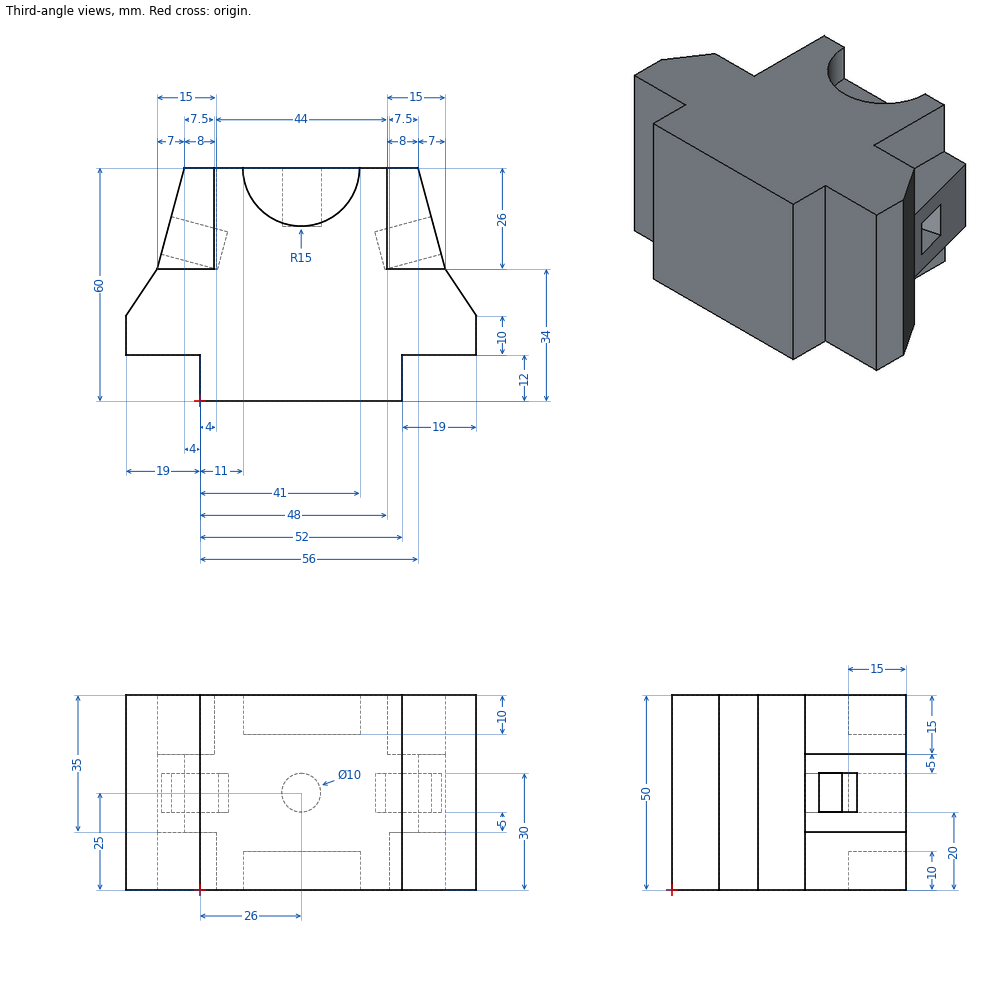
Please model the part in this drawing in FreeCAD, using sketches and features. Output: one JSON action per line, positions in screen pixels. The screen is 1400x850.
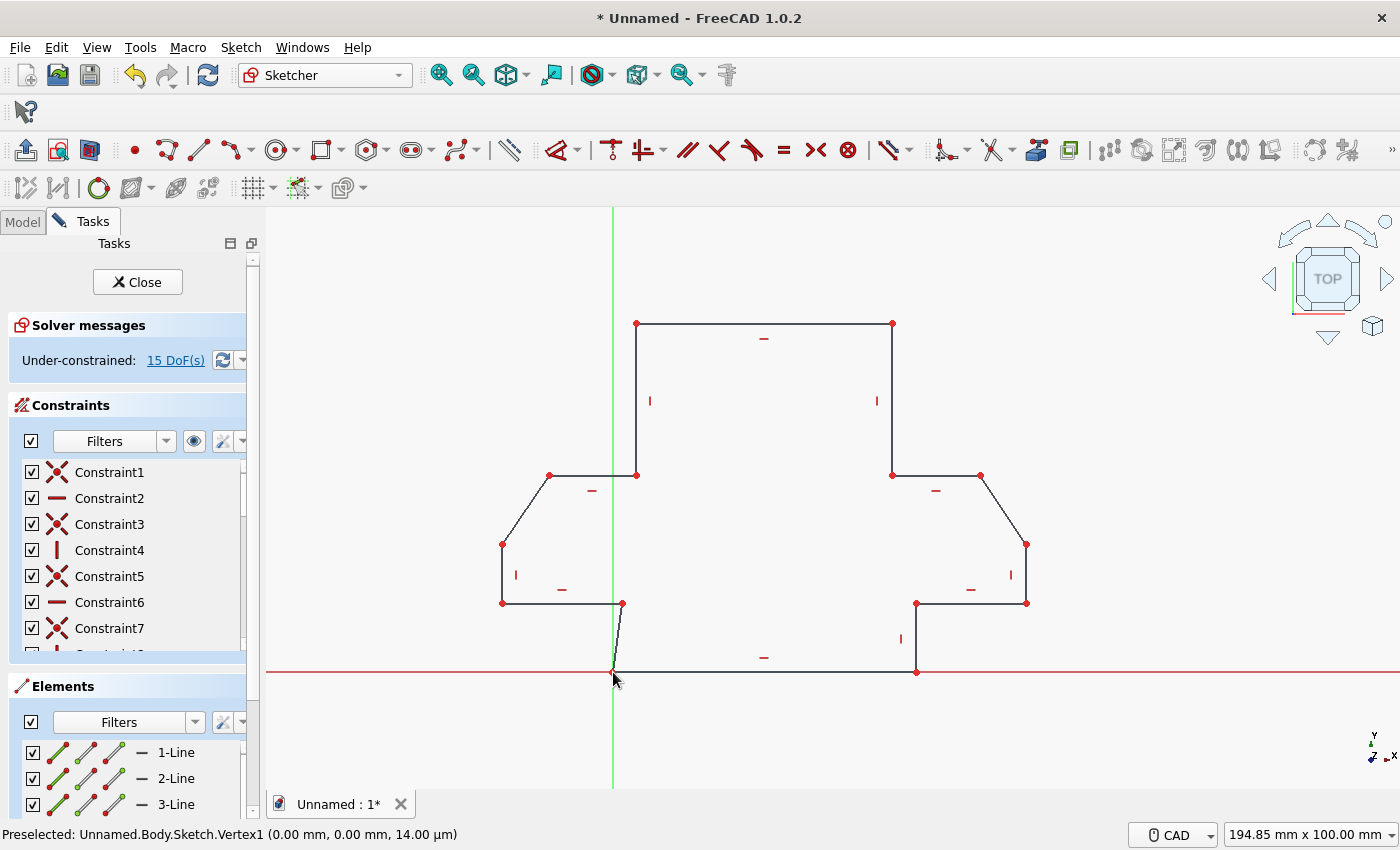
{"action": "left_click", "coordinate": [616, 652]}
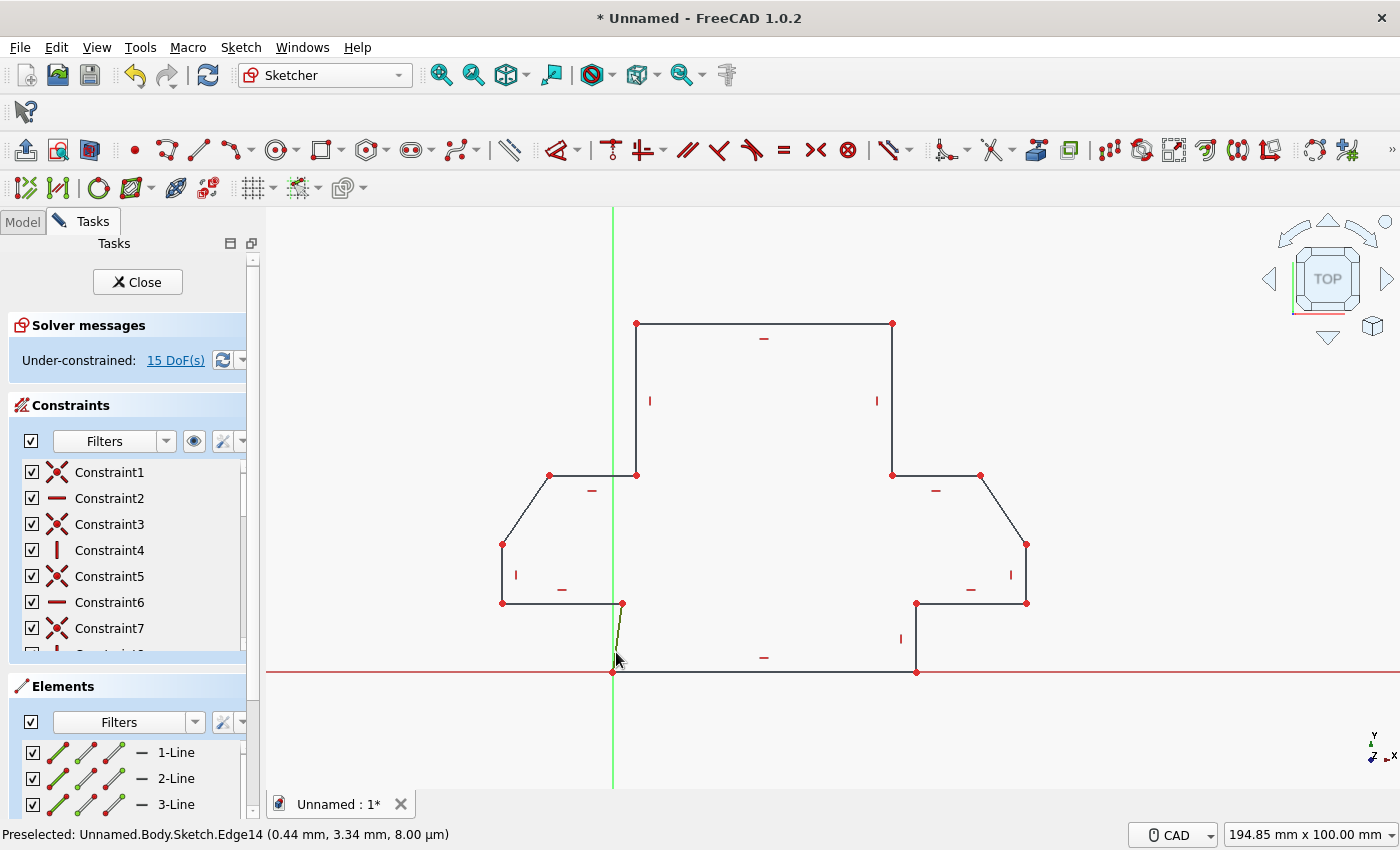
{"action": "left_click", "coordinate": [666, 150]}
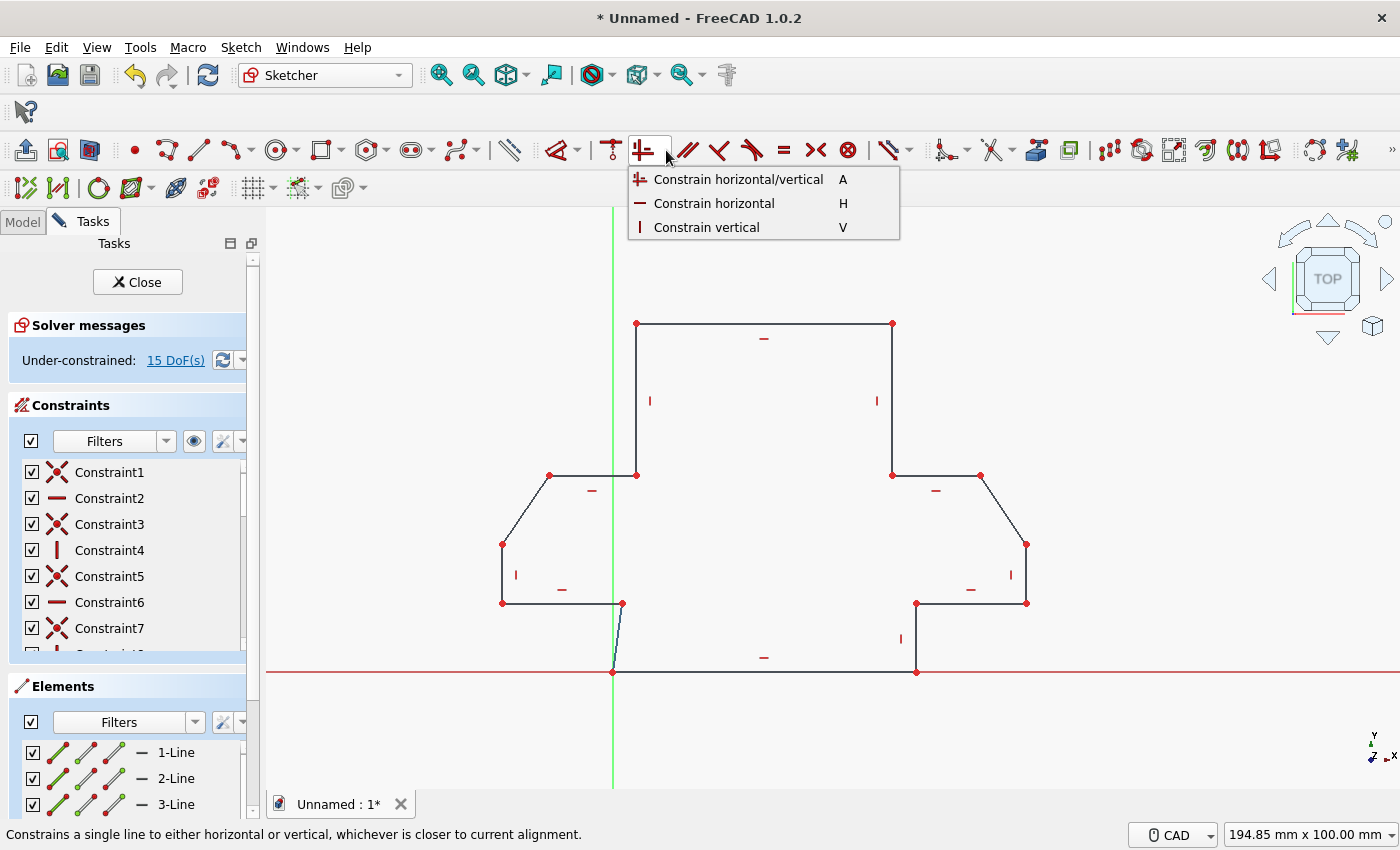
{"action": "left_click", "coordinate": [764, 227]}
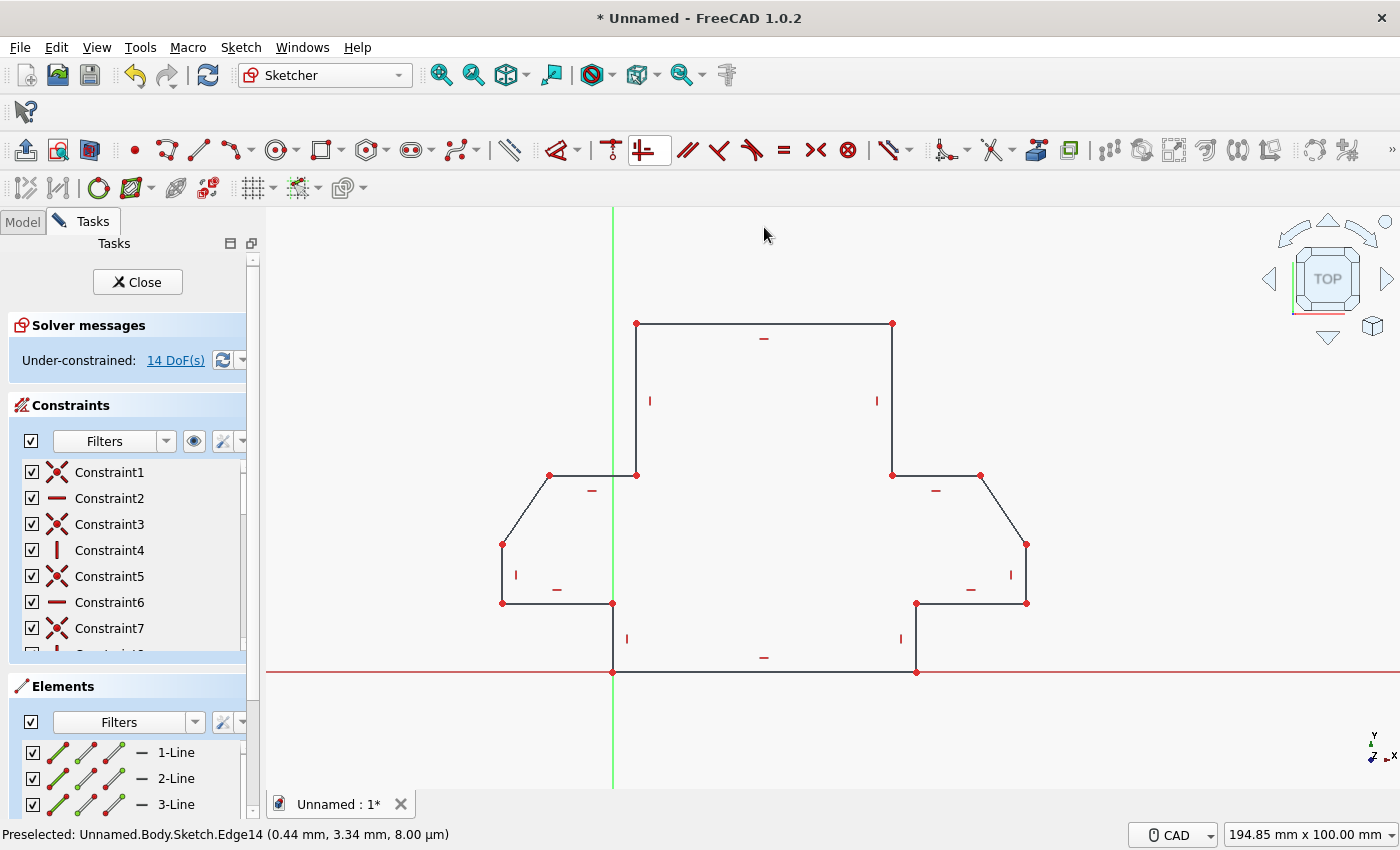
{"action": "left_click", "coordinate": [556, 150]}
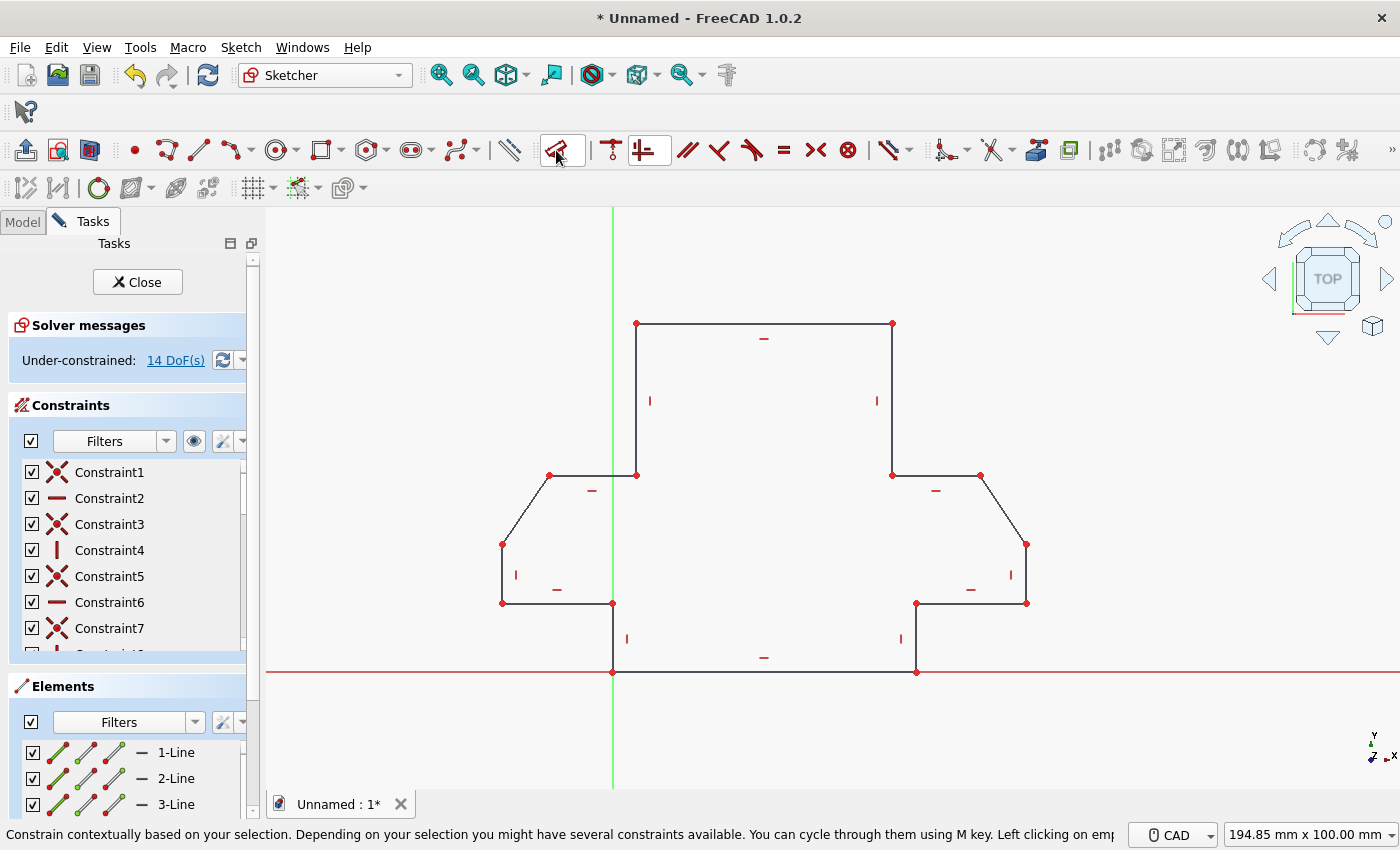
{"action": "left_click", "coordinate": [704, 672]}
{"action": "left_click", "coordinate": [764, 706]}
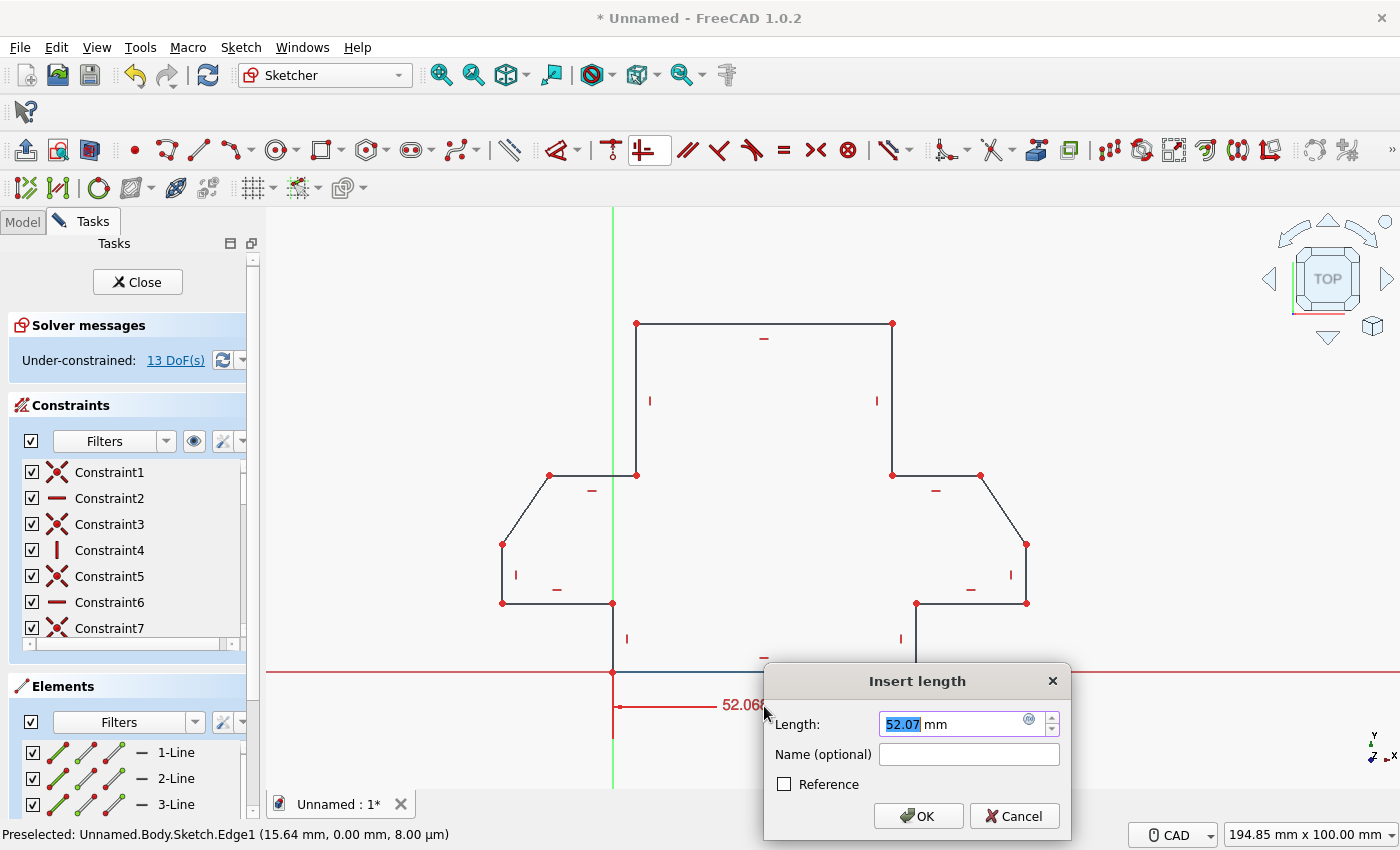
{"action": "type", "text": "52"}
{"action": "key", "text": "Return"}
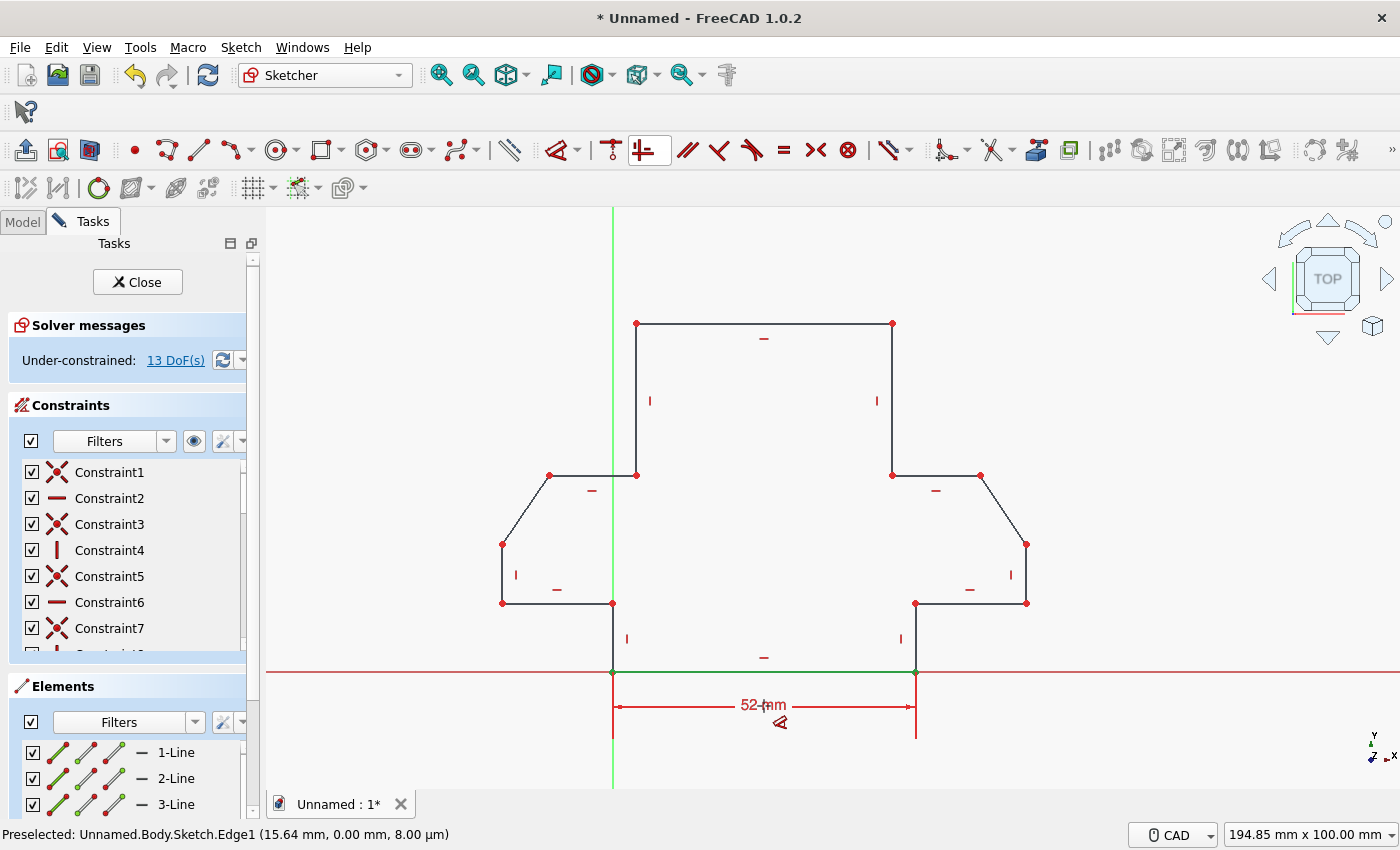
{"action": "left_click", "coordinate": [916, 652]}
{"action": "left_click", "coordinate": [950, 638]}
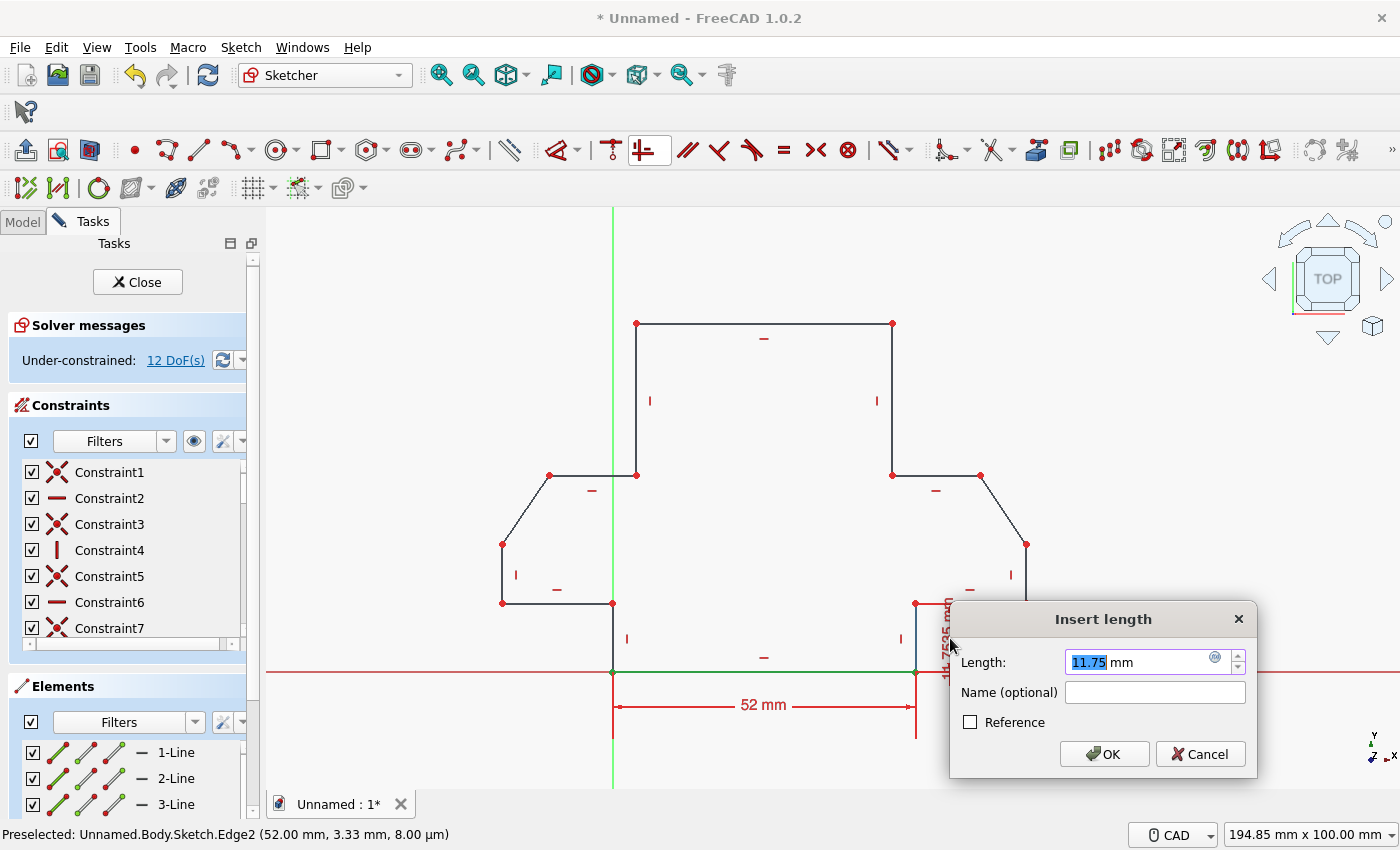
{"action": "type", "text": "12"}
{"action": "key", "text": "Return"}